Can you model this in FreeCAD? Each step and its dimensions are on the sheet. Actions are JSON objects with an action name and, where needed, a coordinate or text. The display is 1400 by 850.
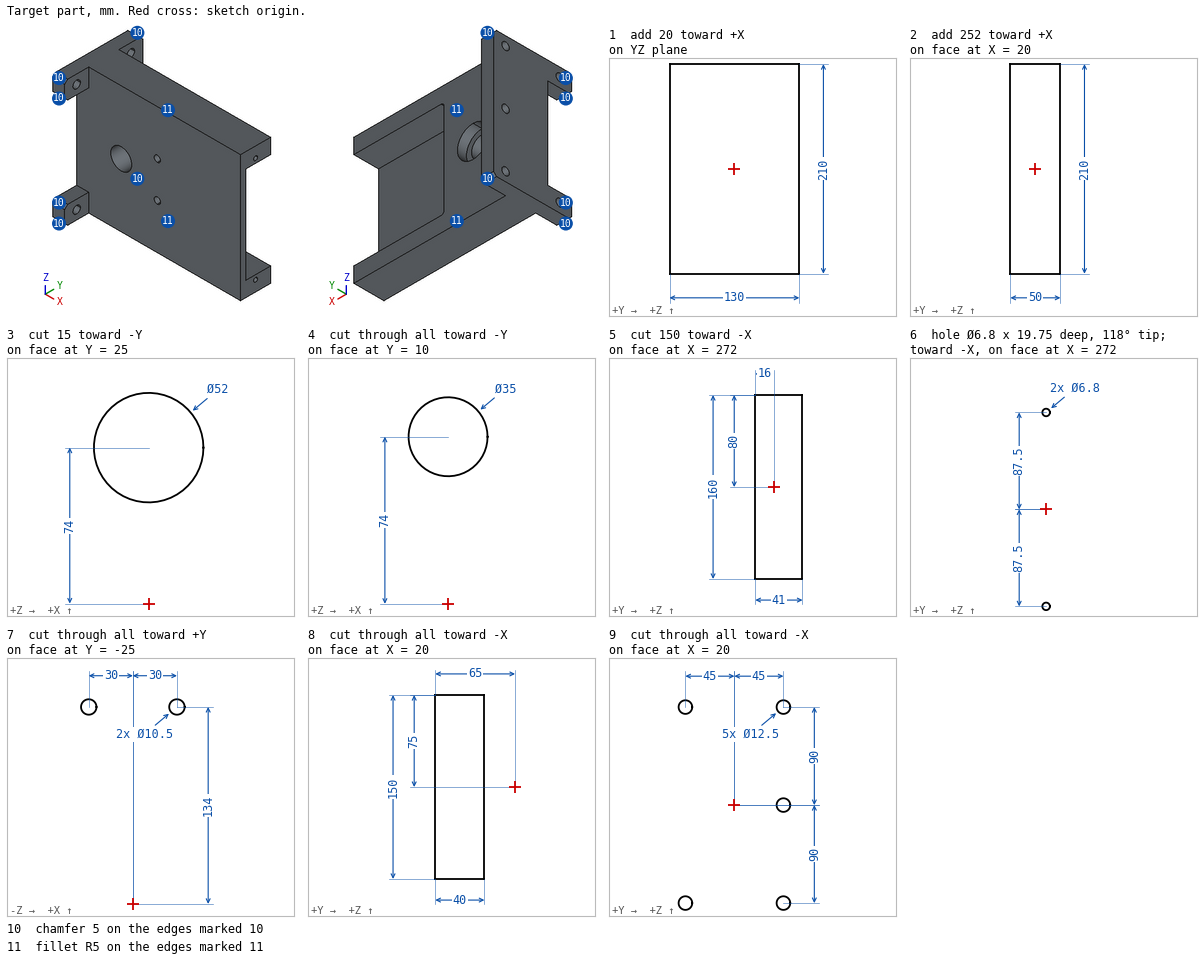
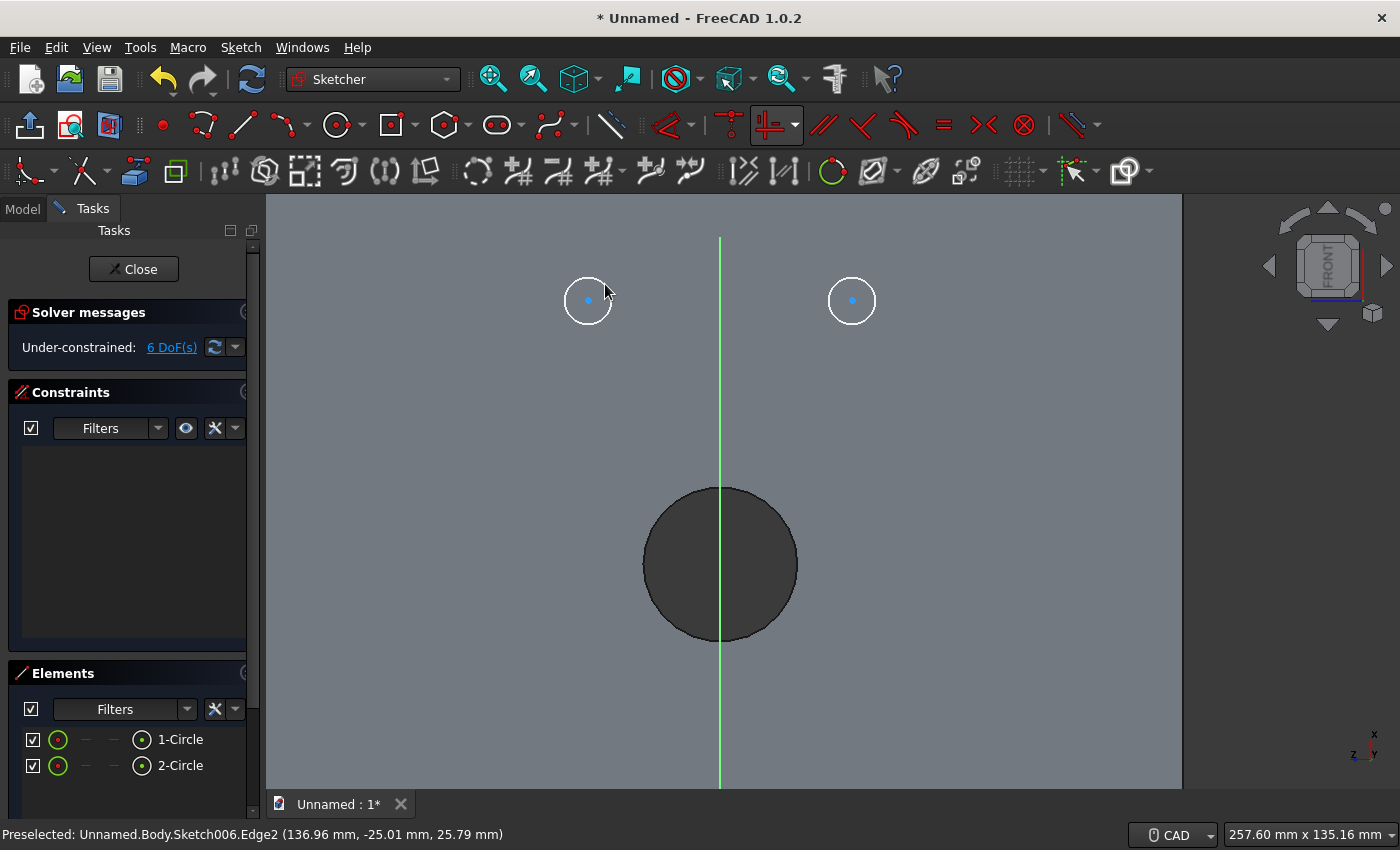
{"action": "left_click", "coordinate": [868, 284]}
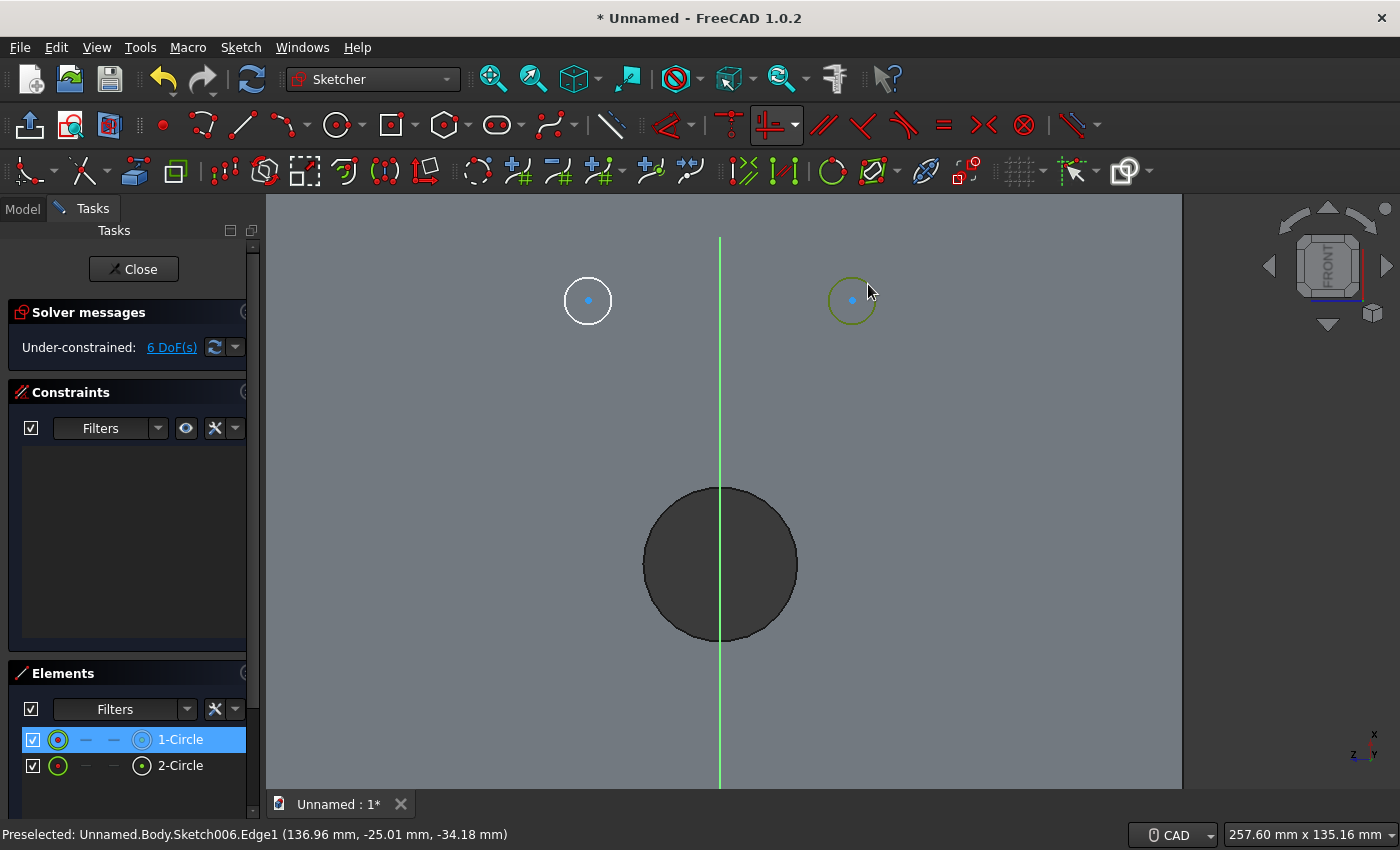
{"action": "left_click", "coordinate": [604, 284]}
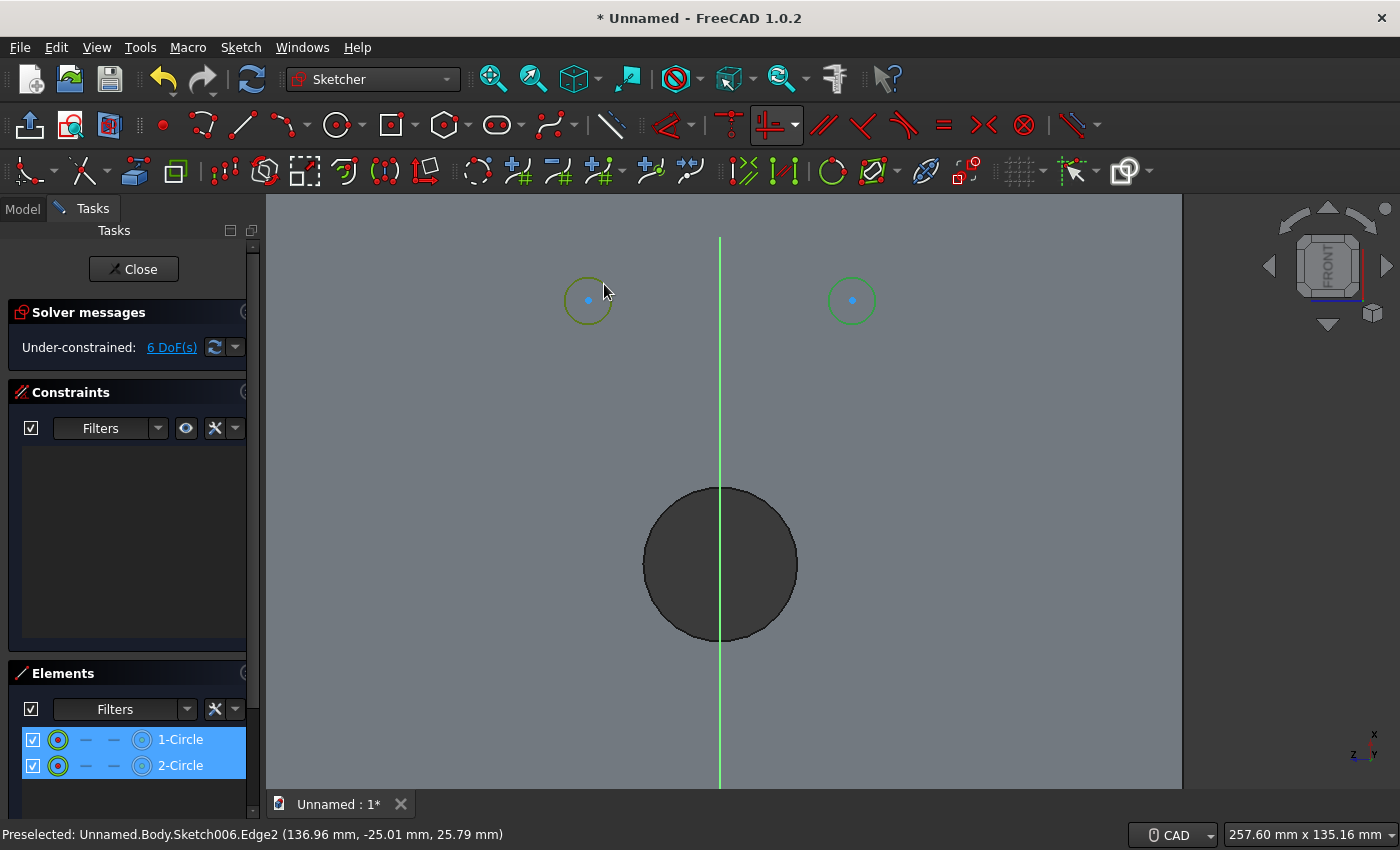
{"action": "left_click", "coordinate": [944, 126]}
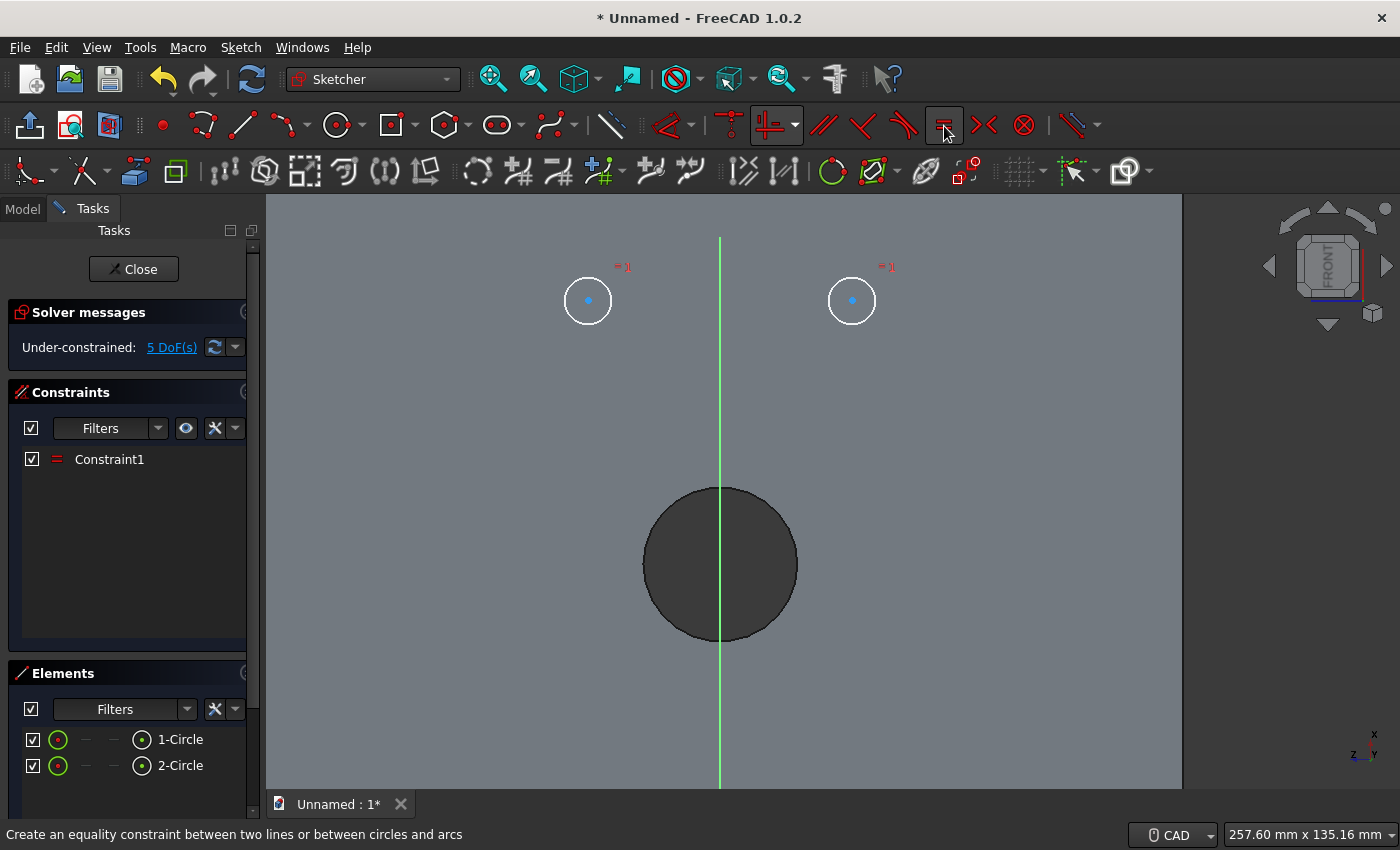
{"action": "left_click", "coordinate": [852, 301]}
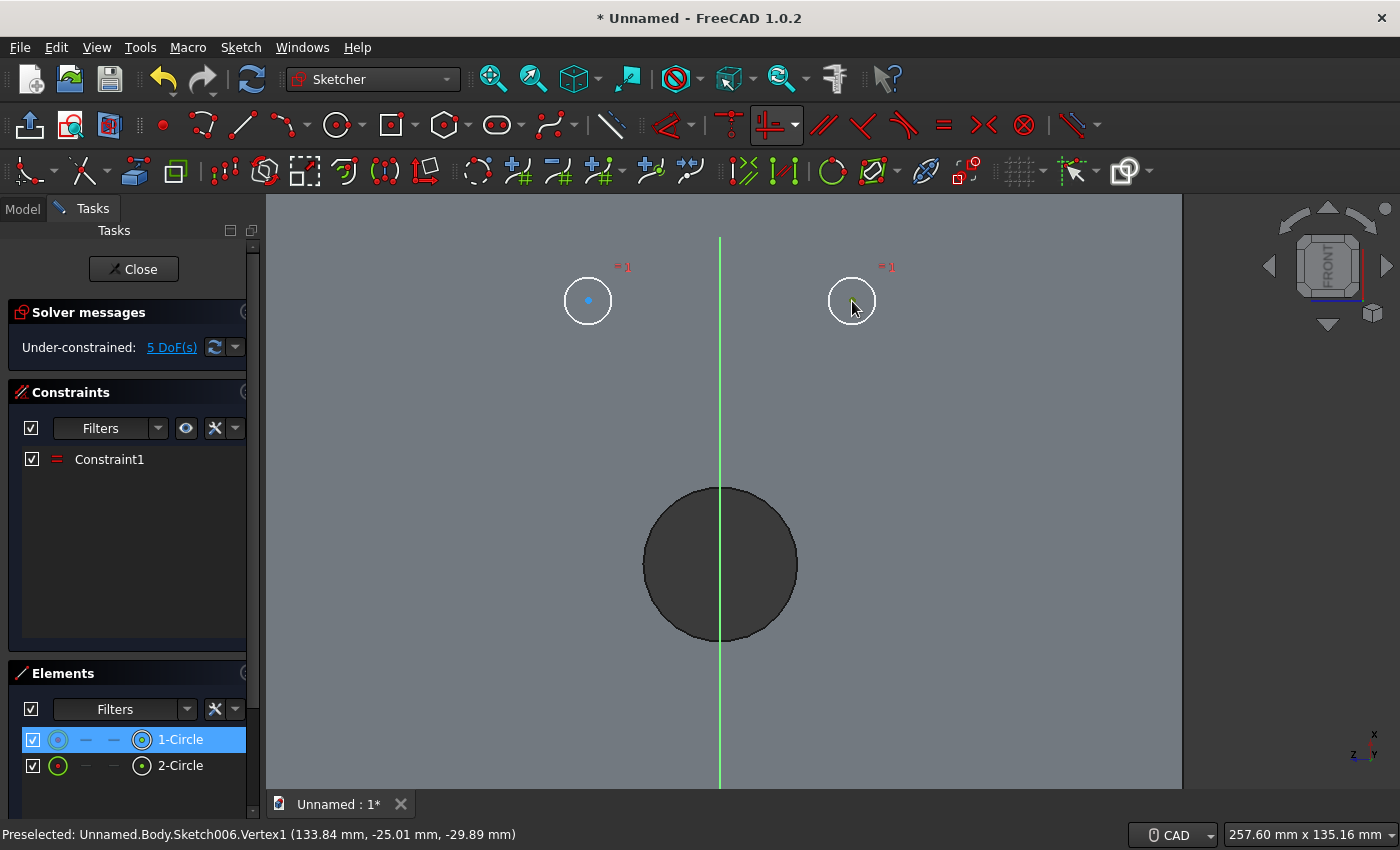
{"action": "left_click", "coordinate": [588, 301]}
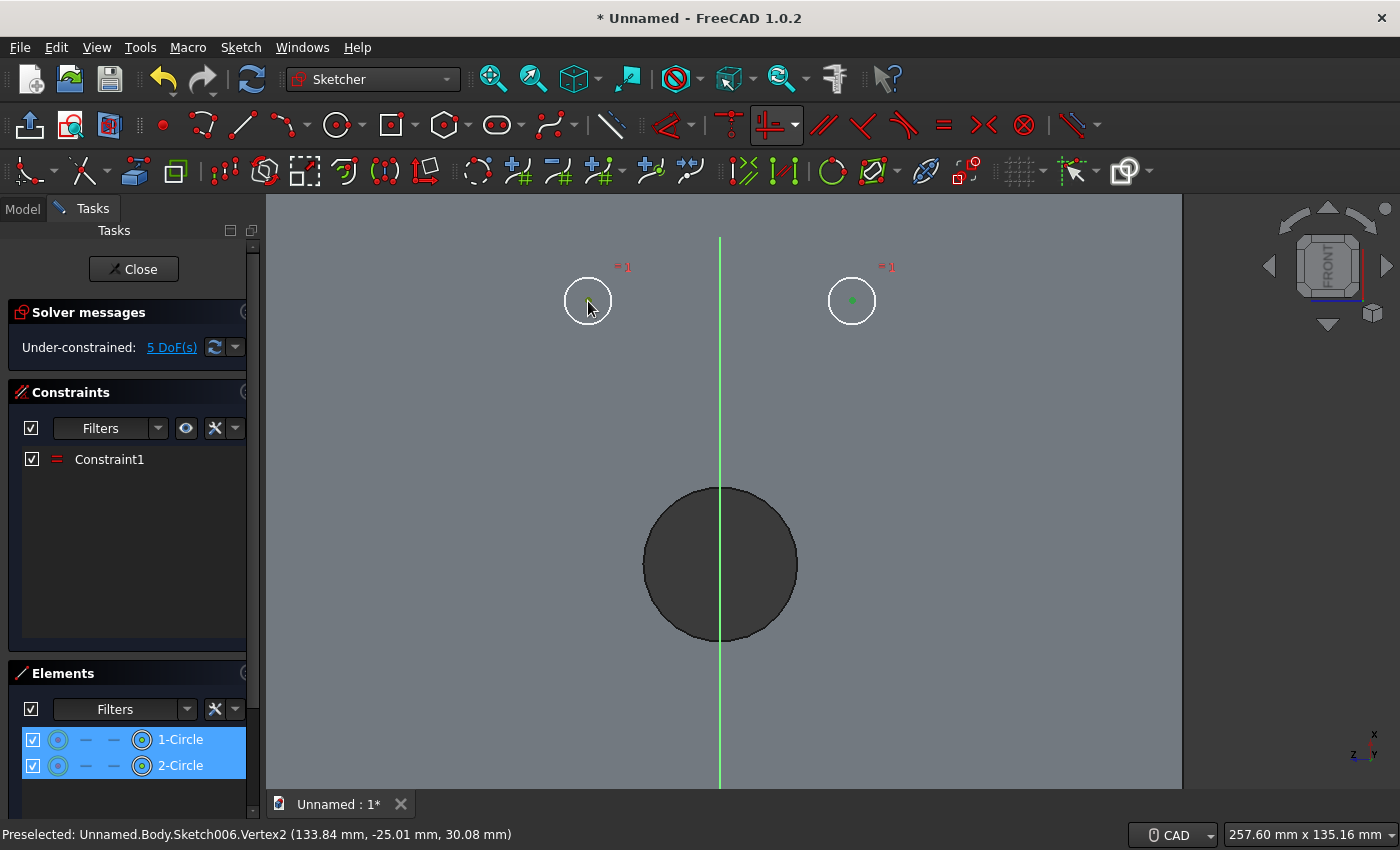
{"action": "left_click", "coordinate": [798, 126]}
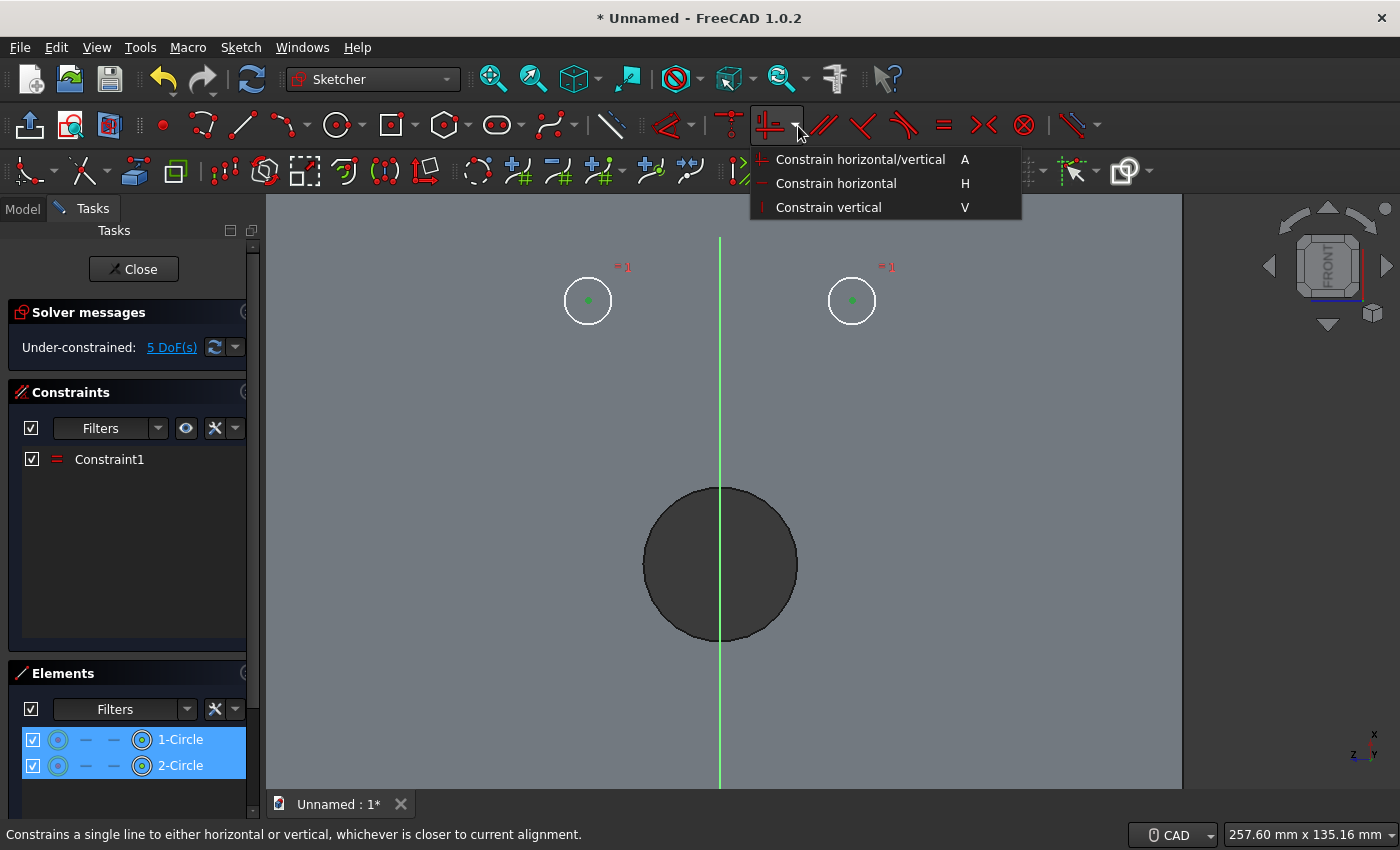
{"action": "left_click", "coordinate": [886, 183]}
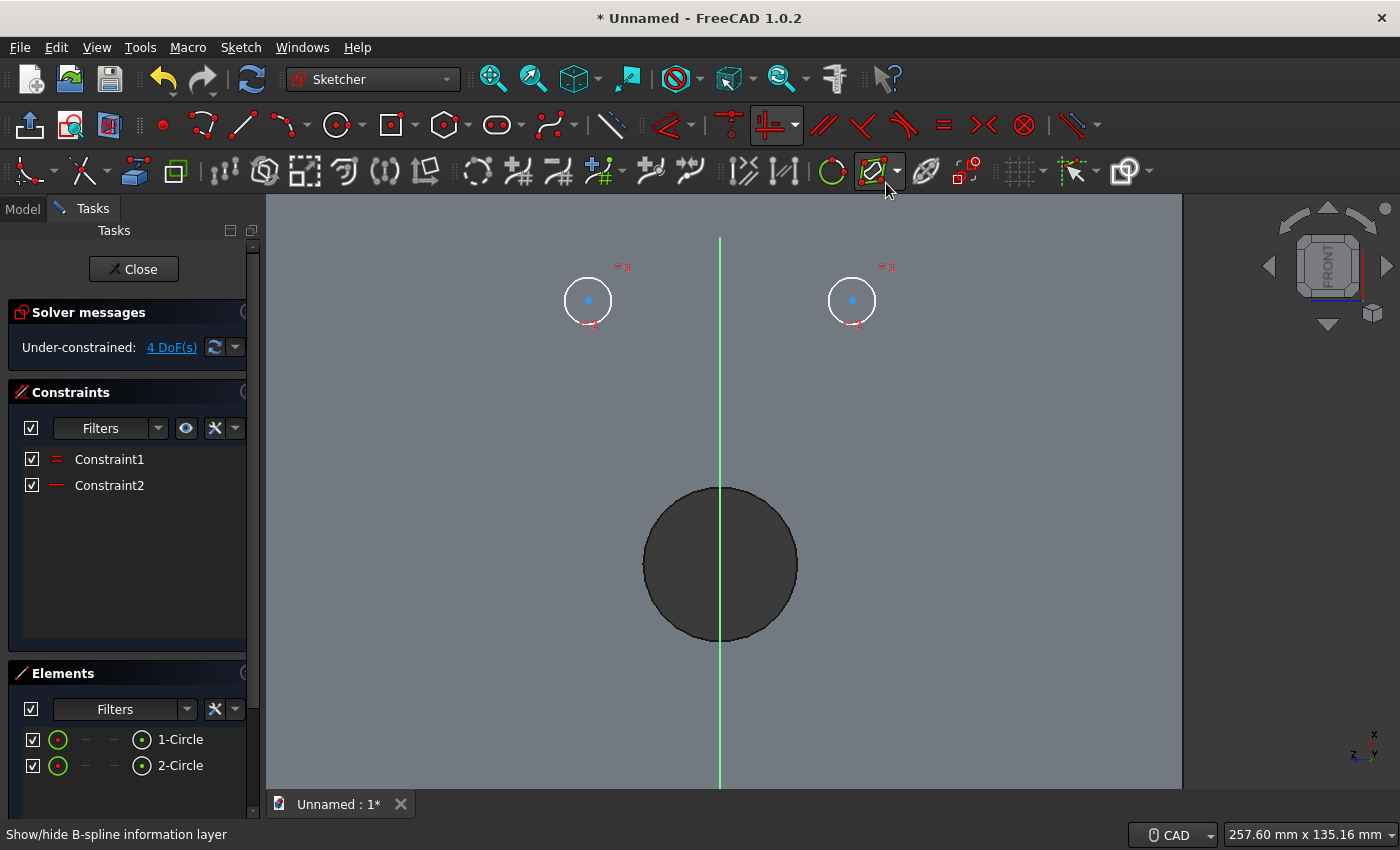
{"action": "left_click", "coordinate": [666, 126]}